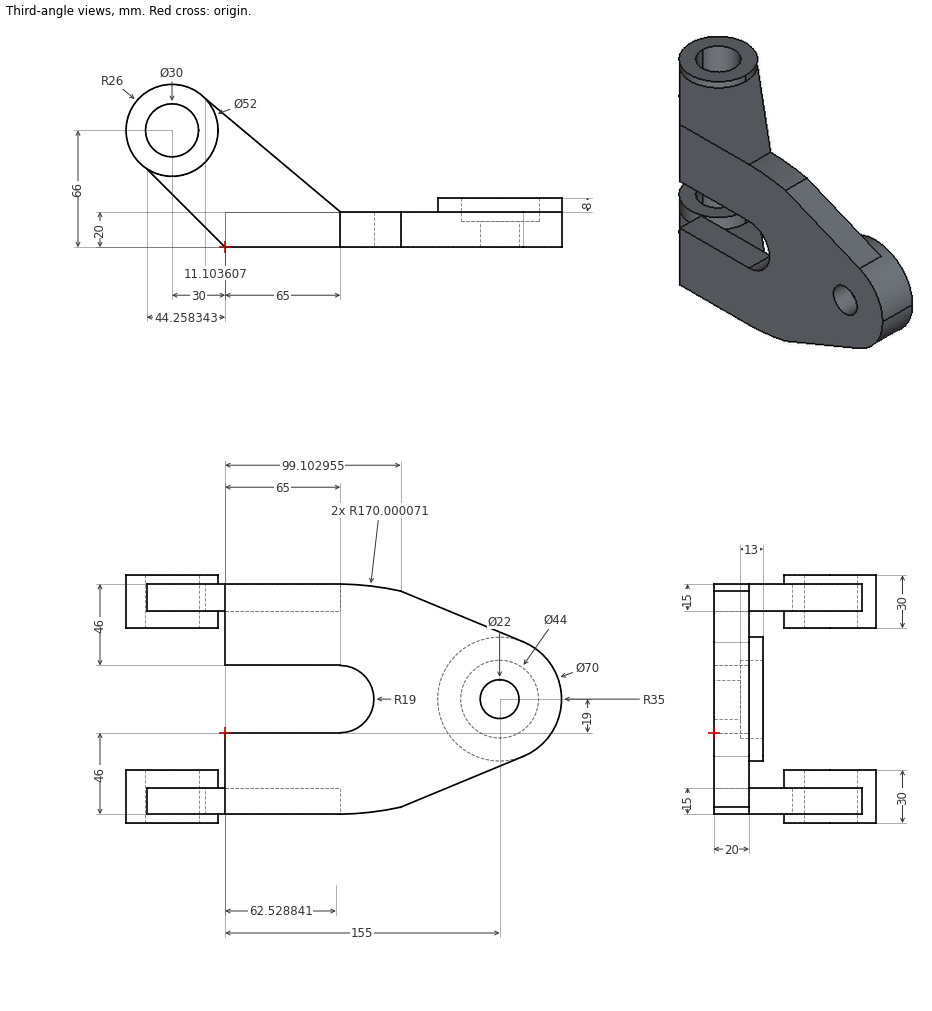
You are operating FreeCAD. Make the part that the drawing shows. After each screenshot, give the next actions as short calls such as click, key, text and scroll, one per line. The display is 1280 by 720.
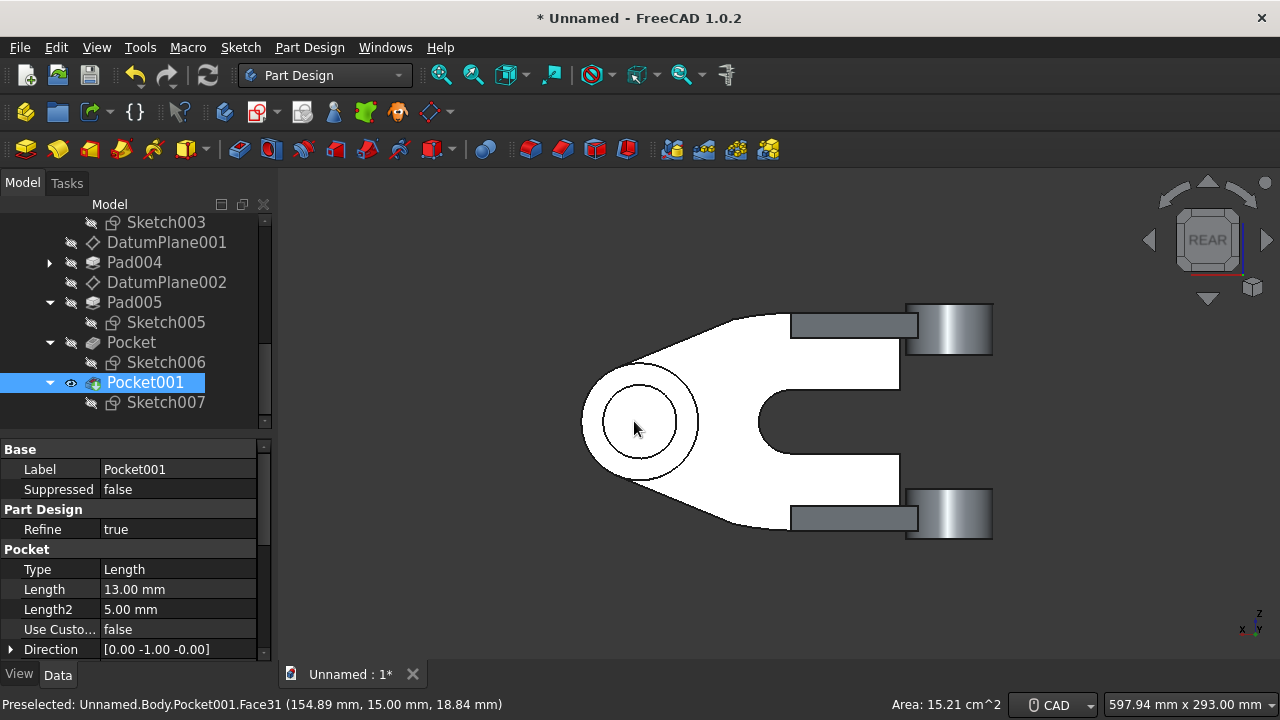
click(258, 112)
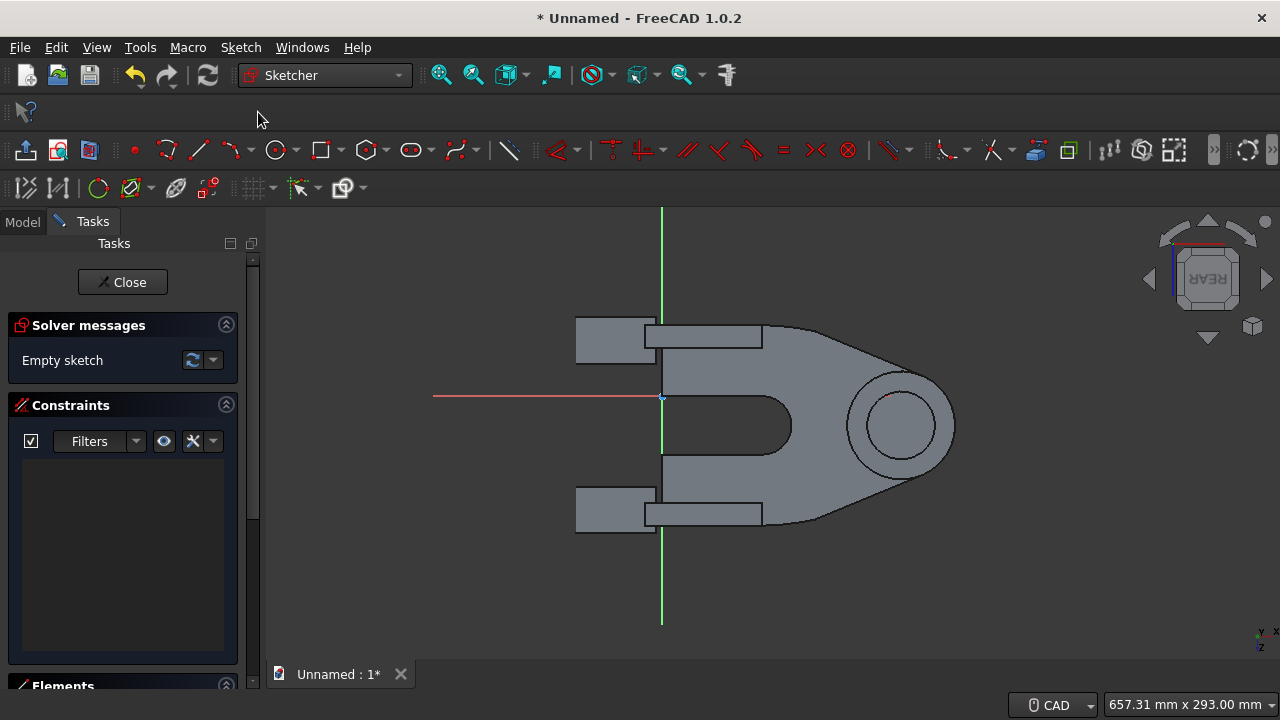
click(90, 150)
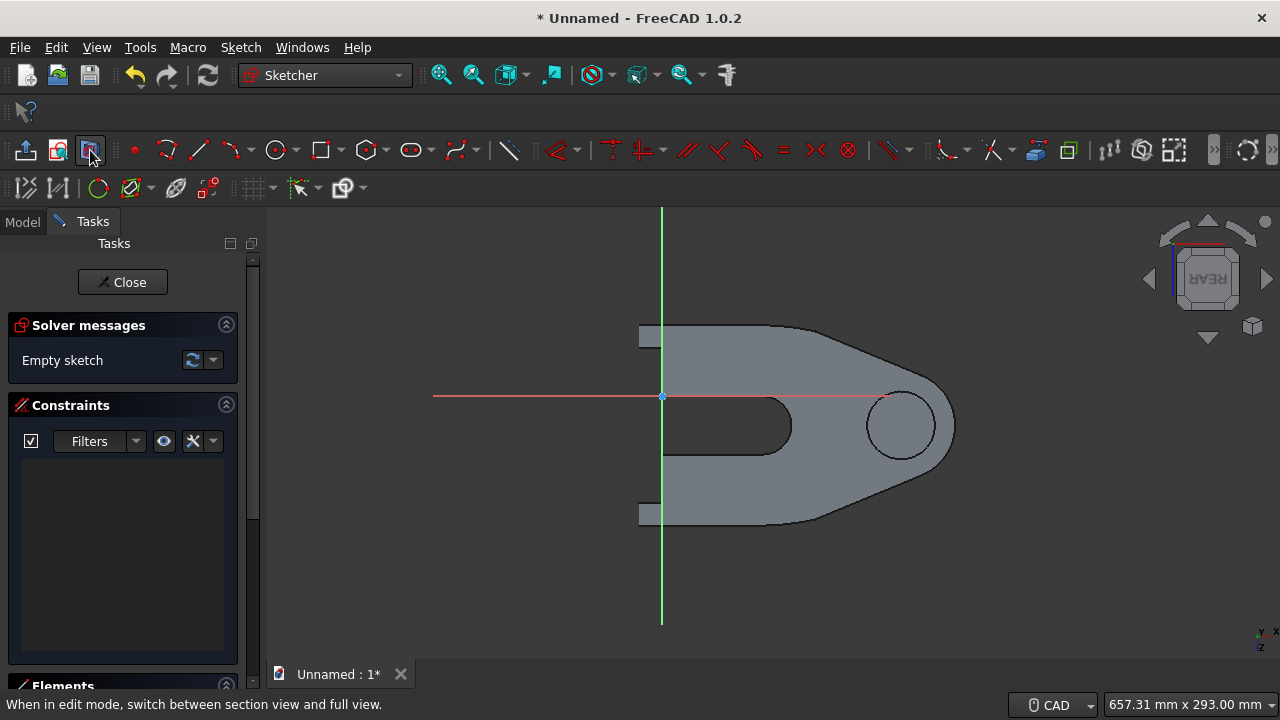
scroll(926, 424, up, 11)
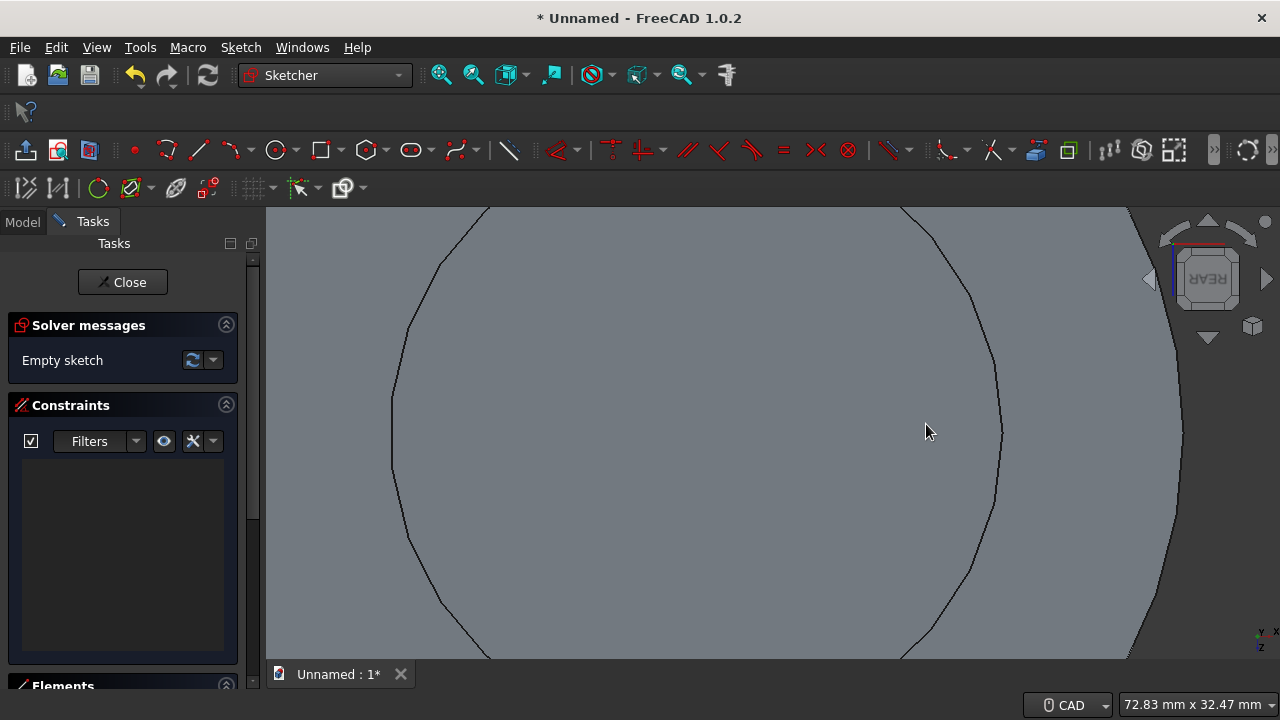
key(g)
key(c)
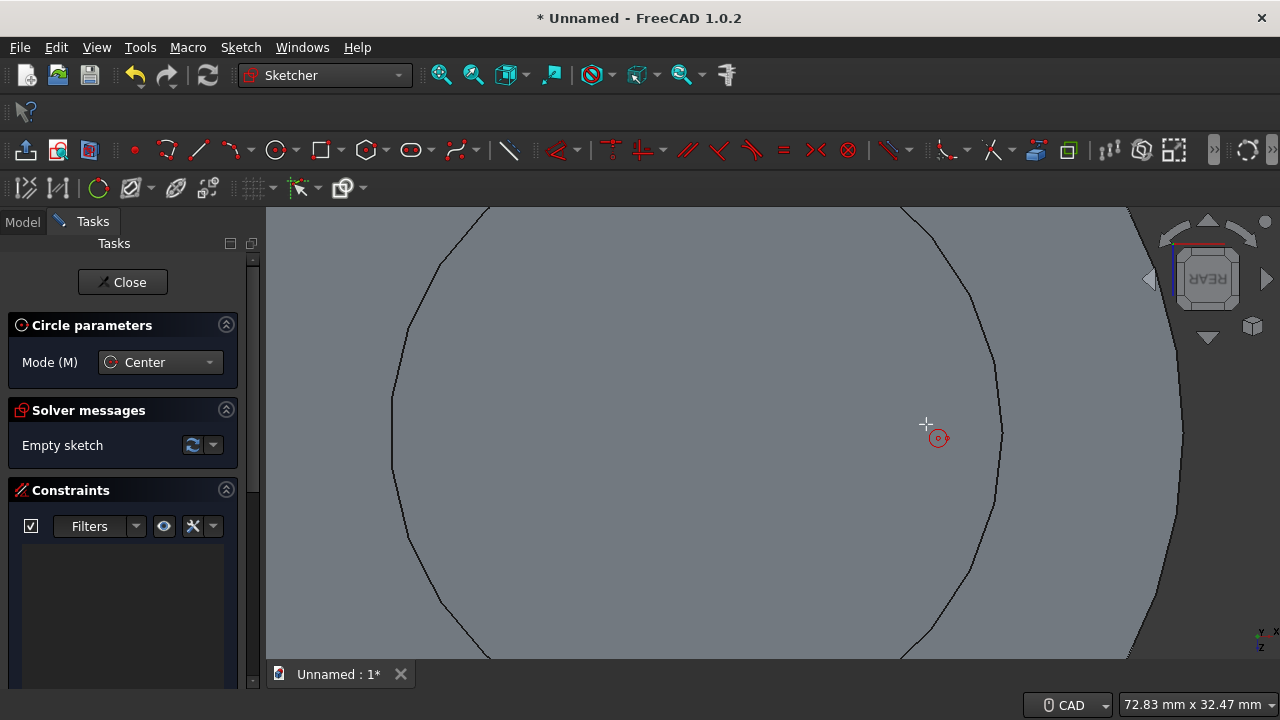
click(696, 433)
move(805, 325)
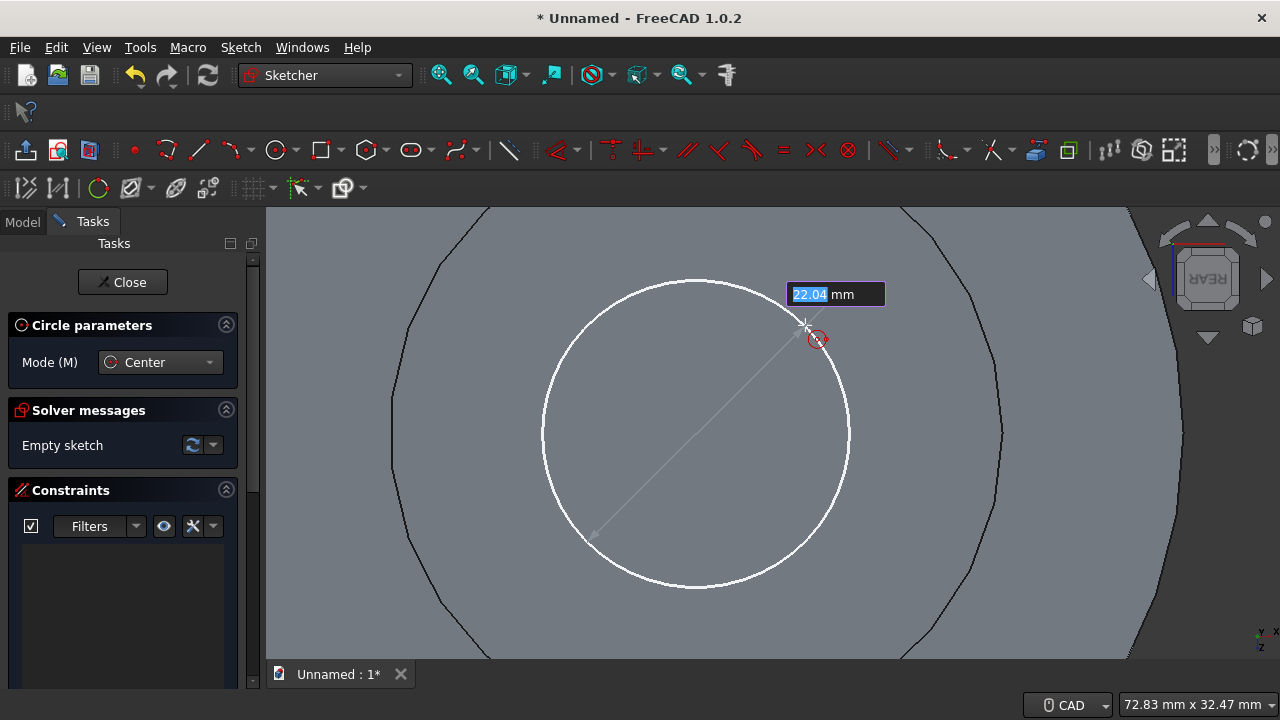
text(22)
key(Return)
key(Escape)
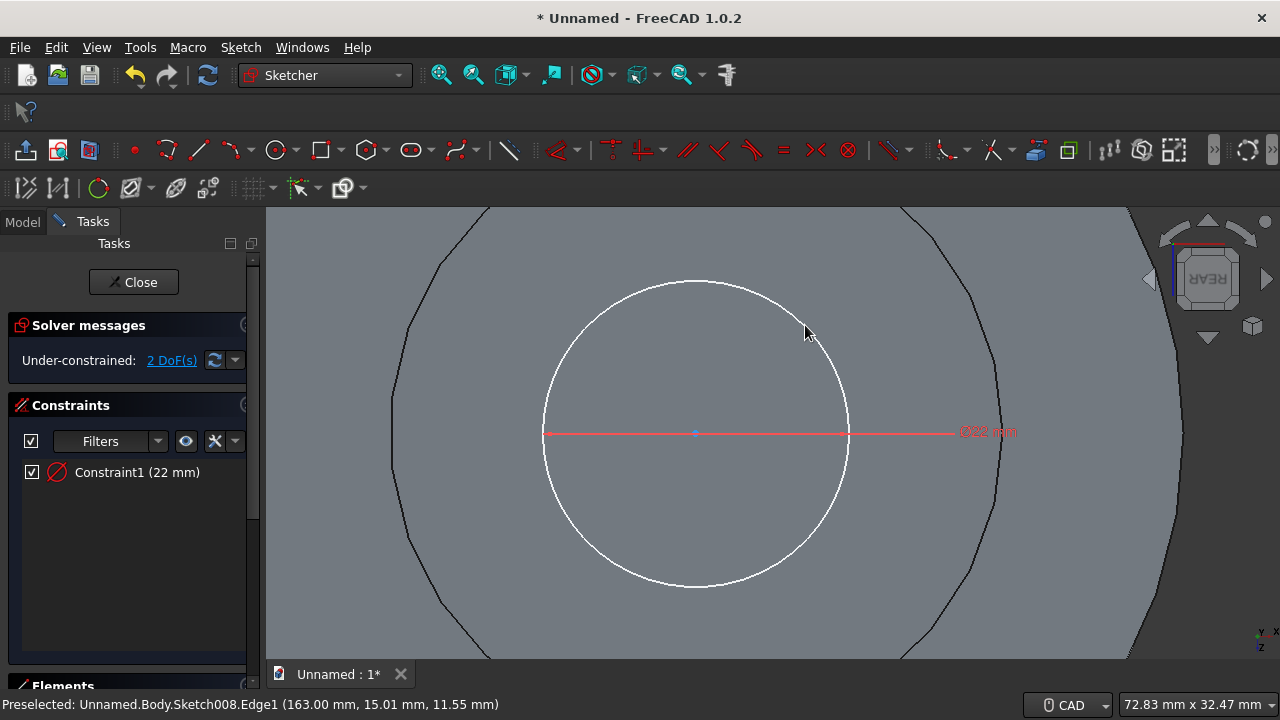
click(556, 150)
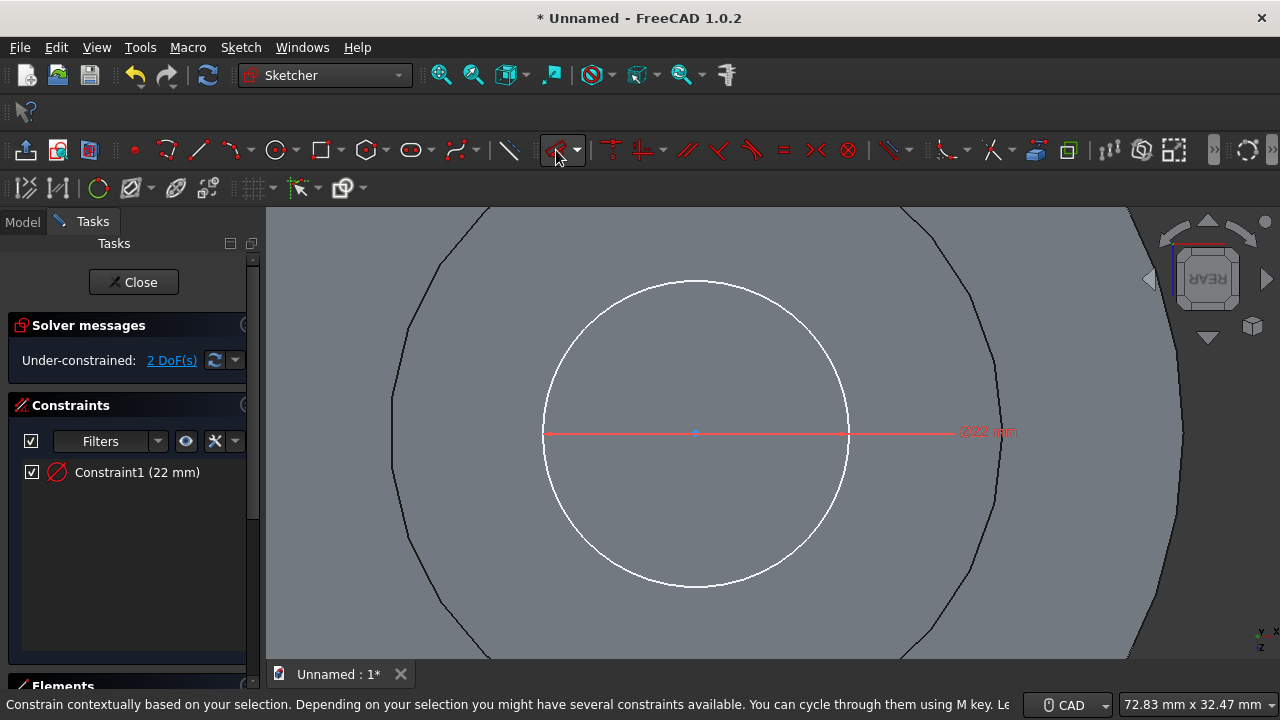
click(696, 434)
click(730, 334)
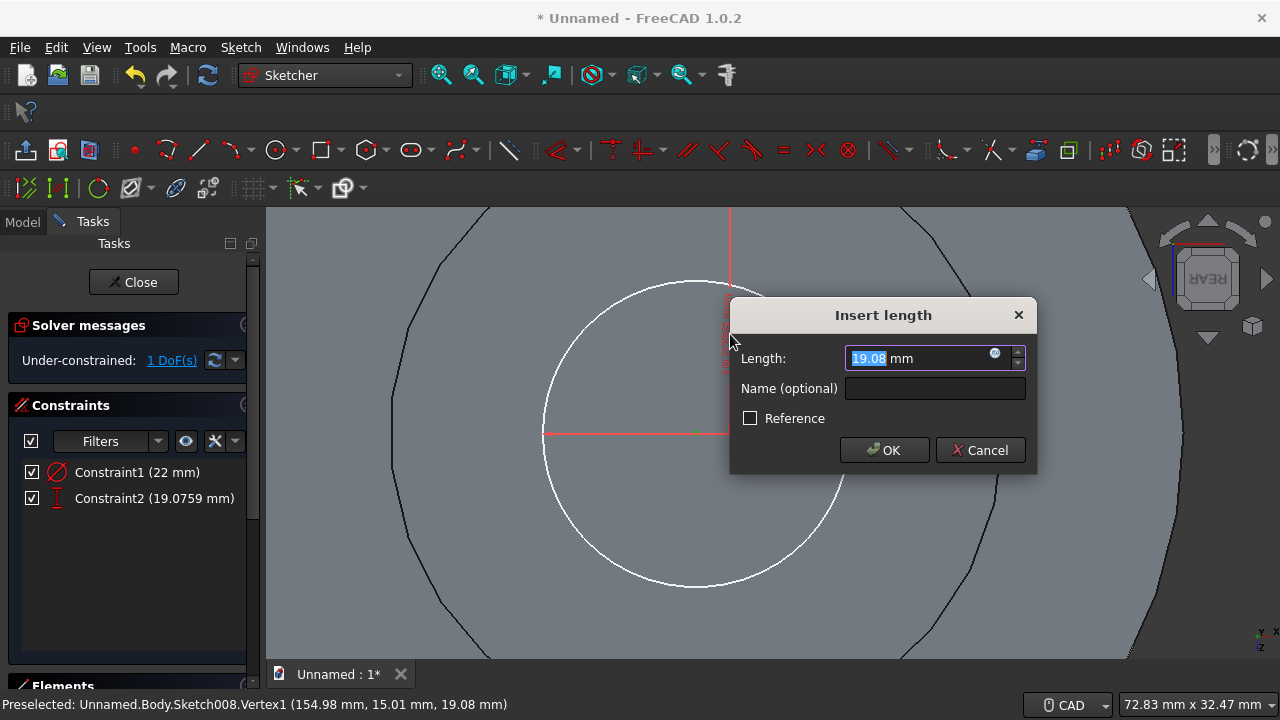
text(19)
key(Return)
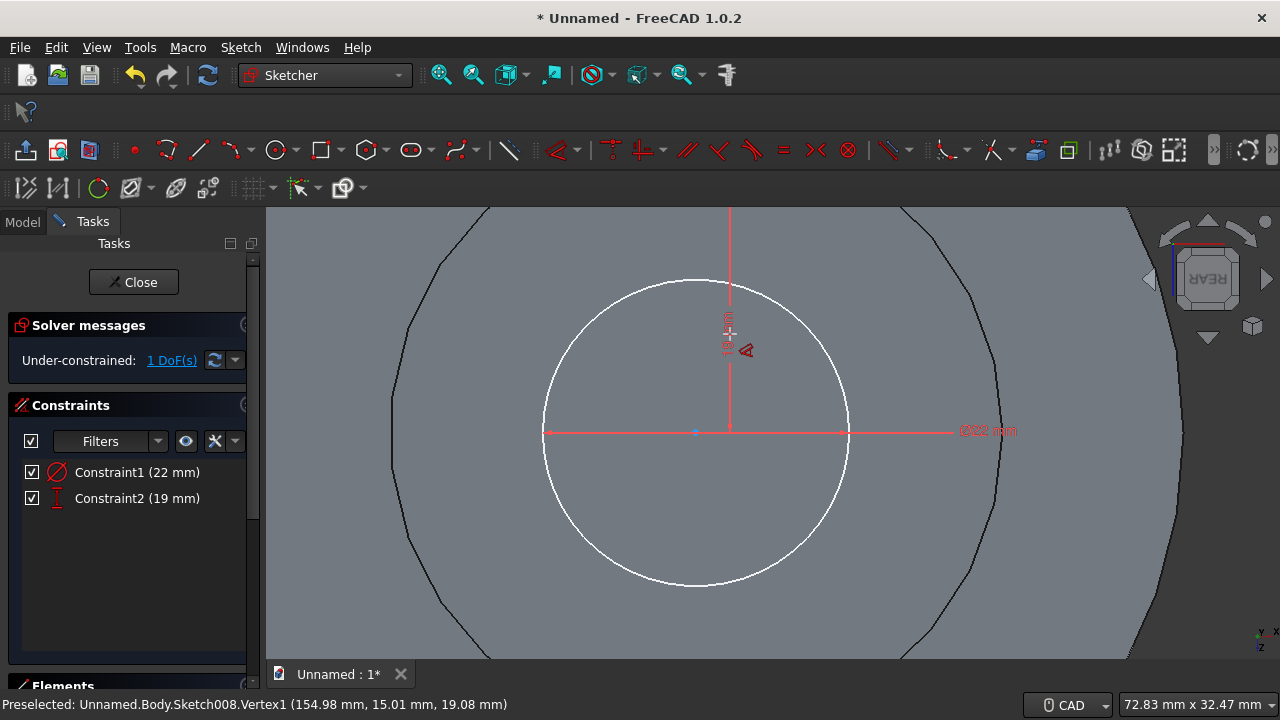
click(696, 433)
click(495, 467)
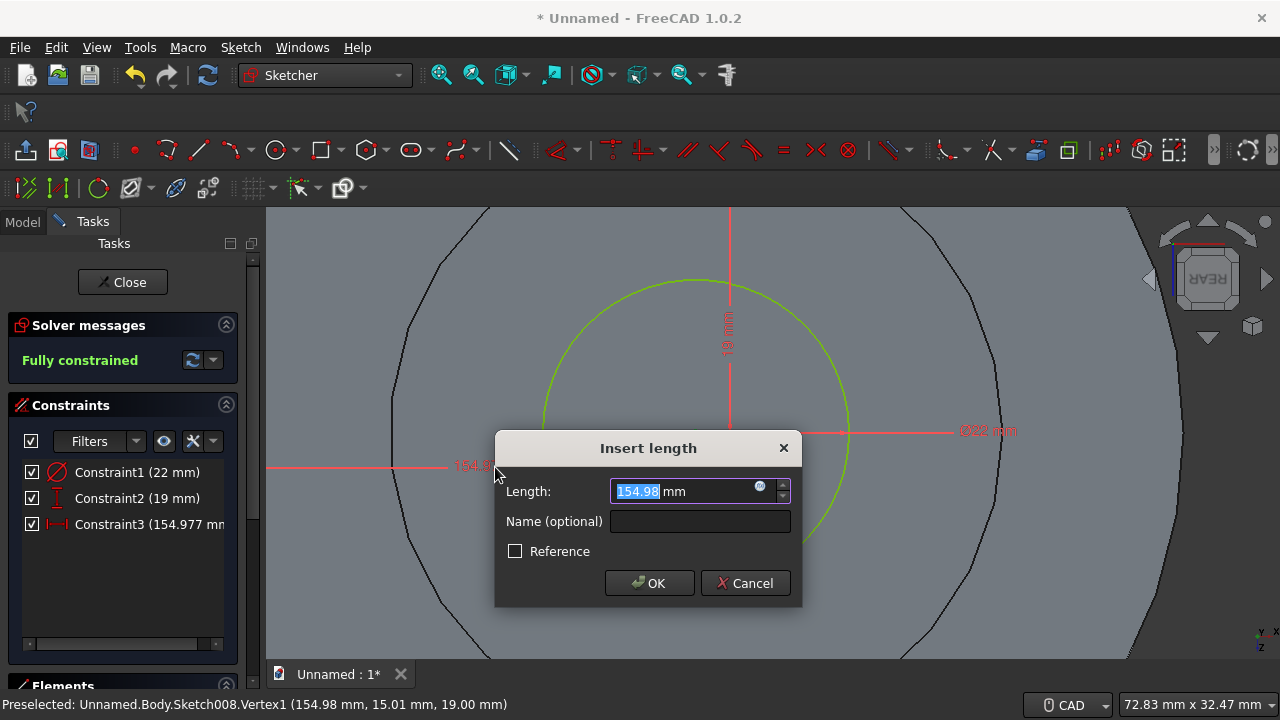
text(155)
key(Return)
key(Escape)